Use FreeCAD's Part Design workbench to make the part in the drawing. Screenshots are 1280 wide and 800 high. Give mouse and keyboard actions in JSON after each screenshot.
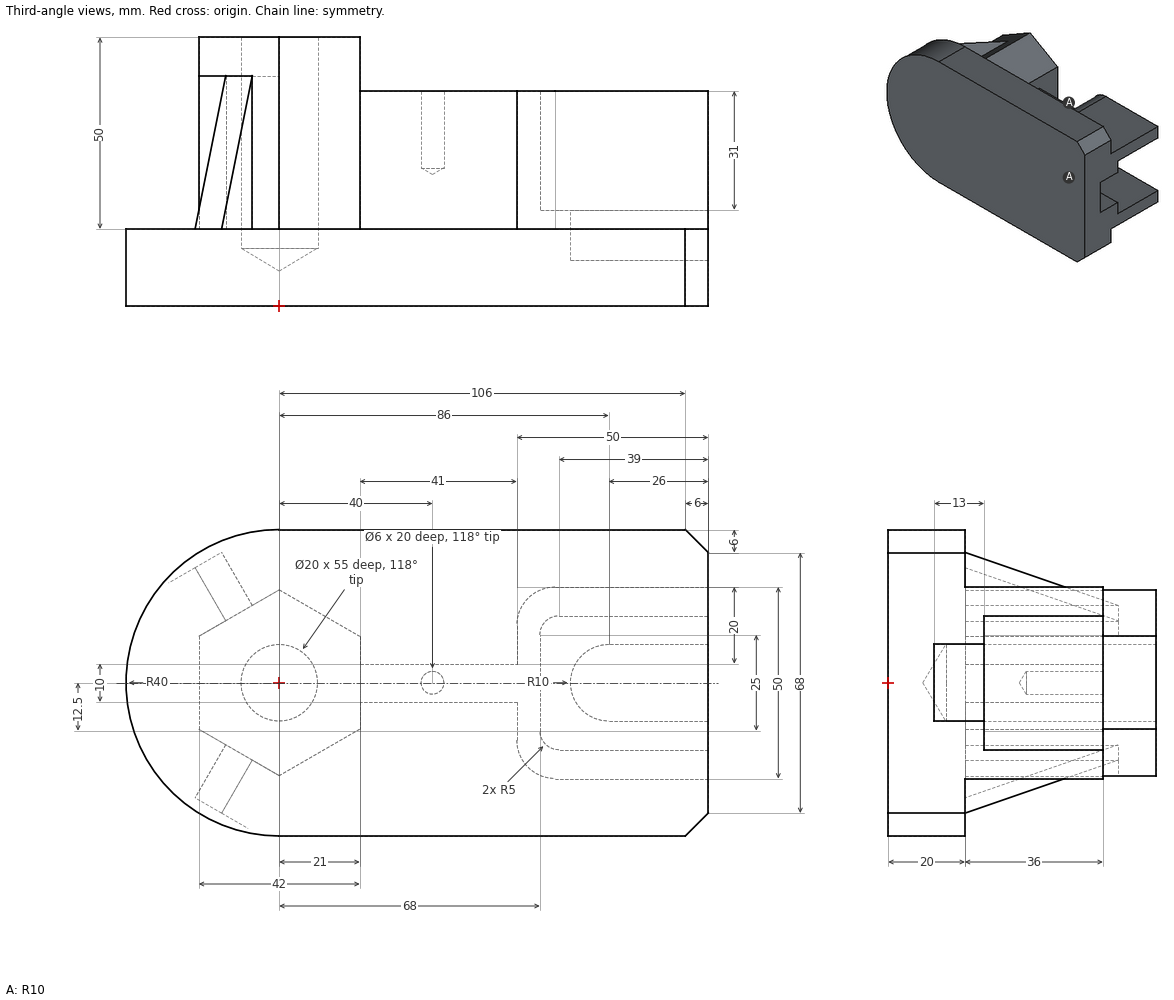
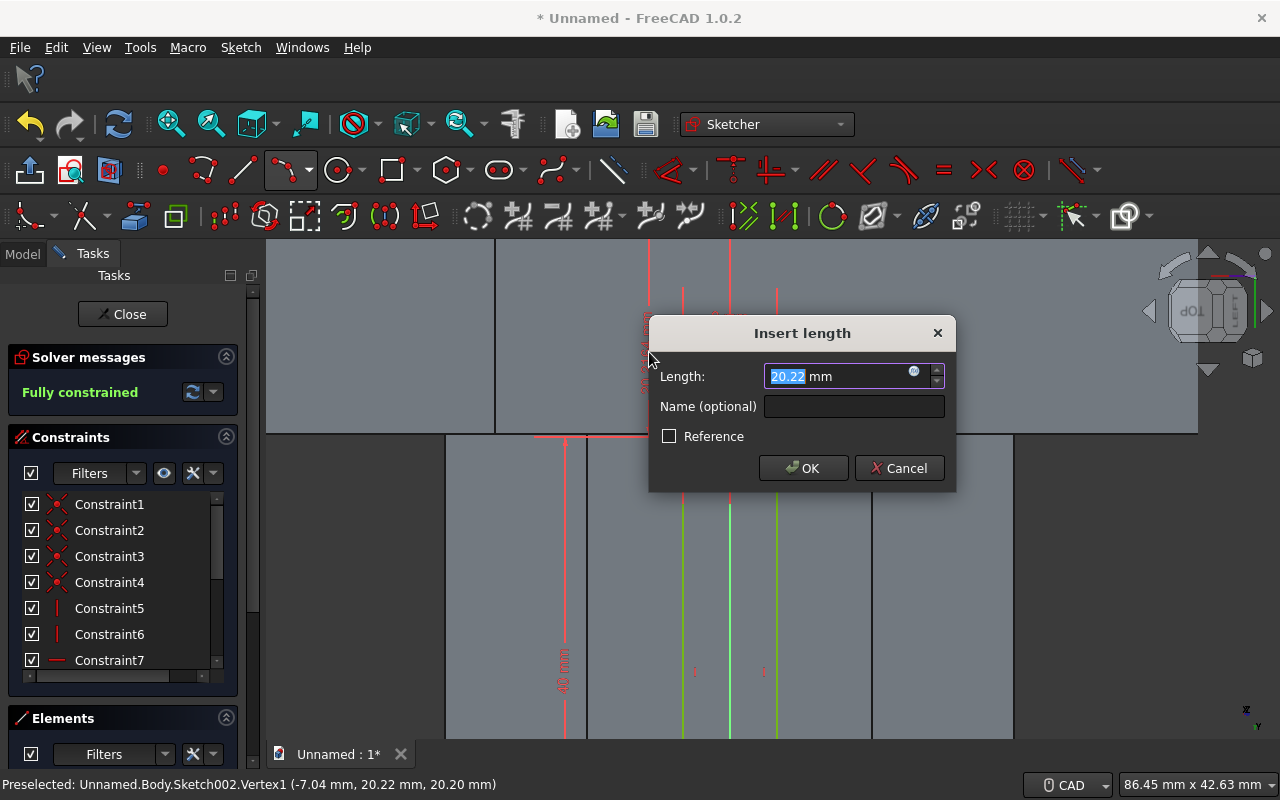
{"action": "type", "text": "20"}
{"action": "key", "text": "Return"}
{"action": "key", "text": "Escape"}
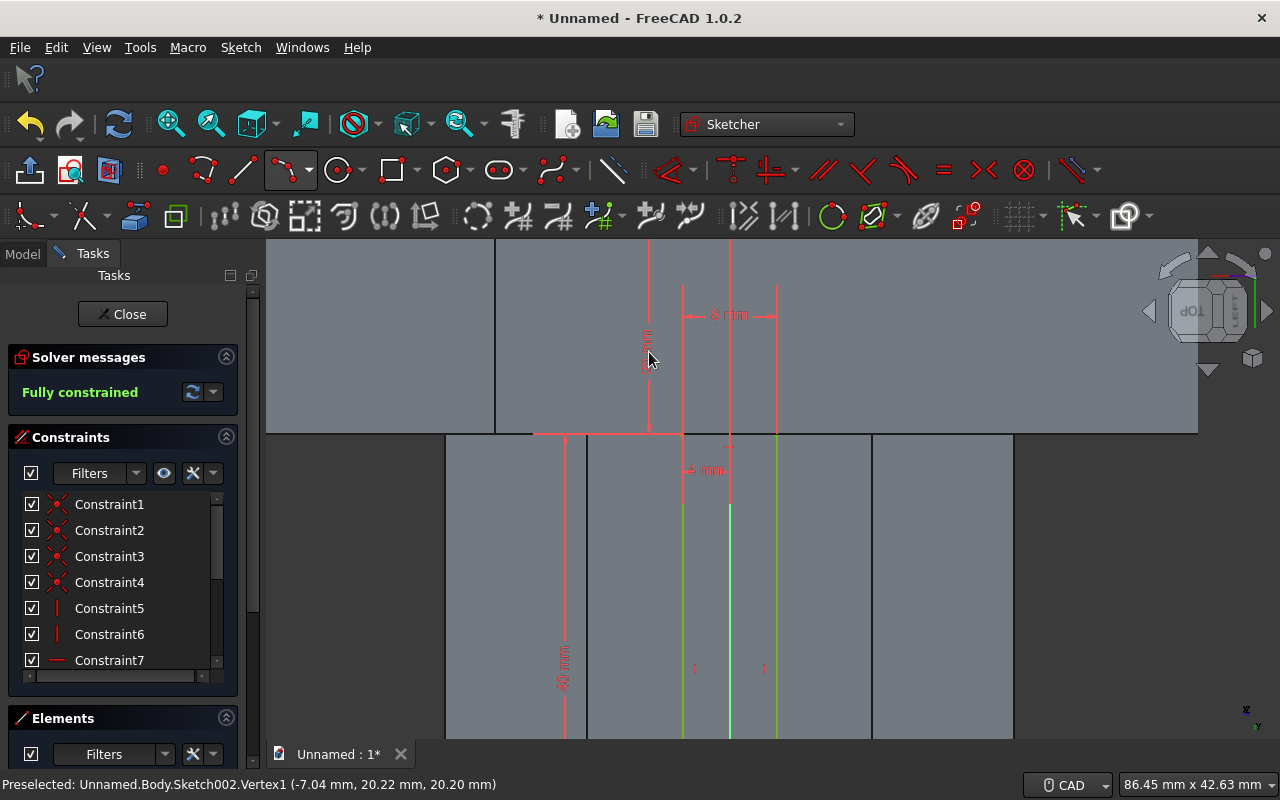
{"action": "left_click", "coordinate": [123, 314]}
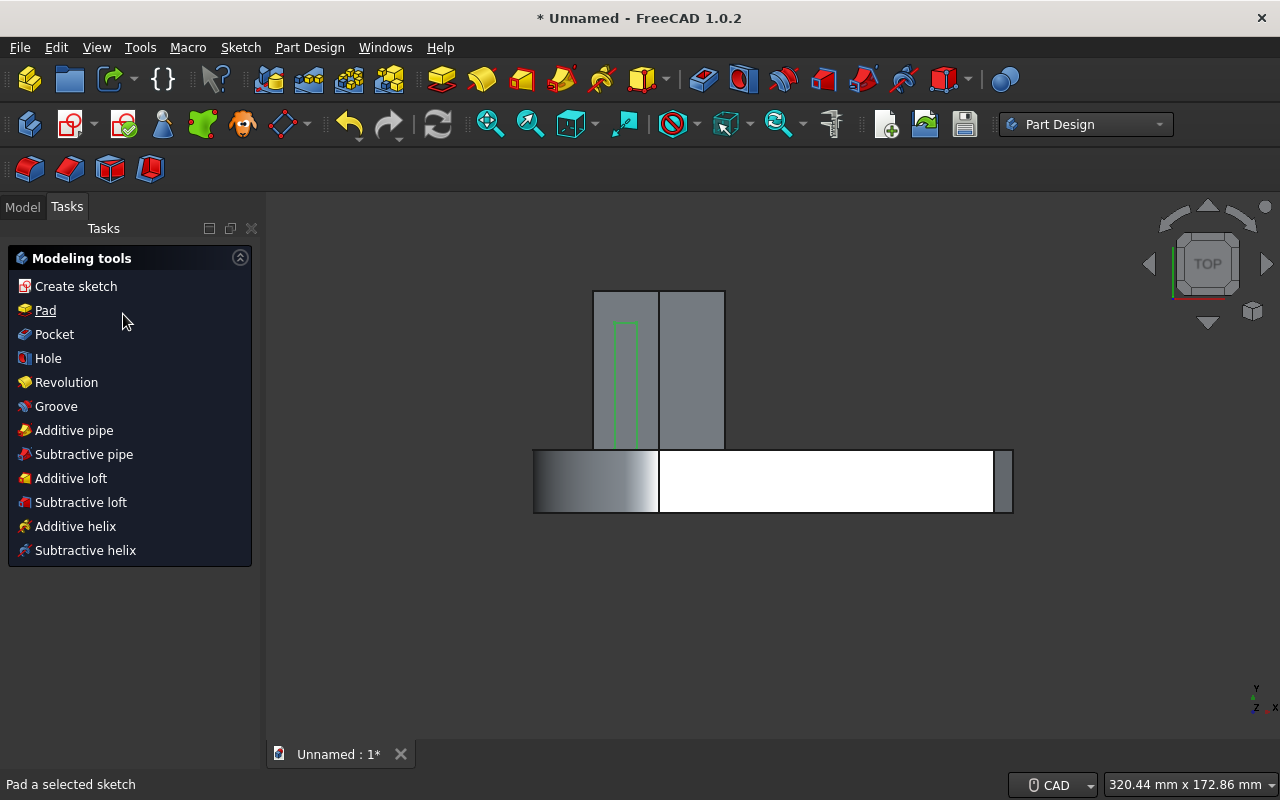
{"action": "left_click", "coordinate": [442, 80]}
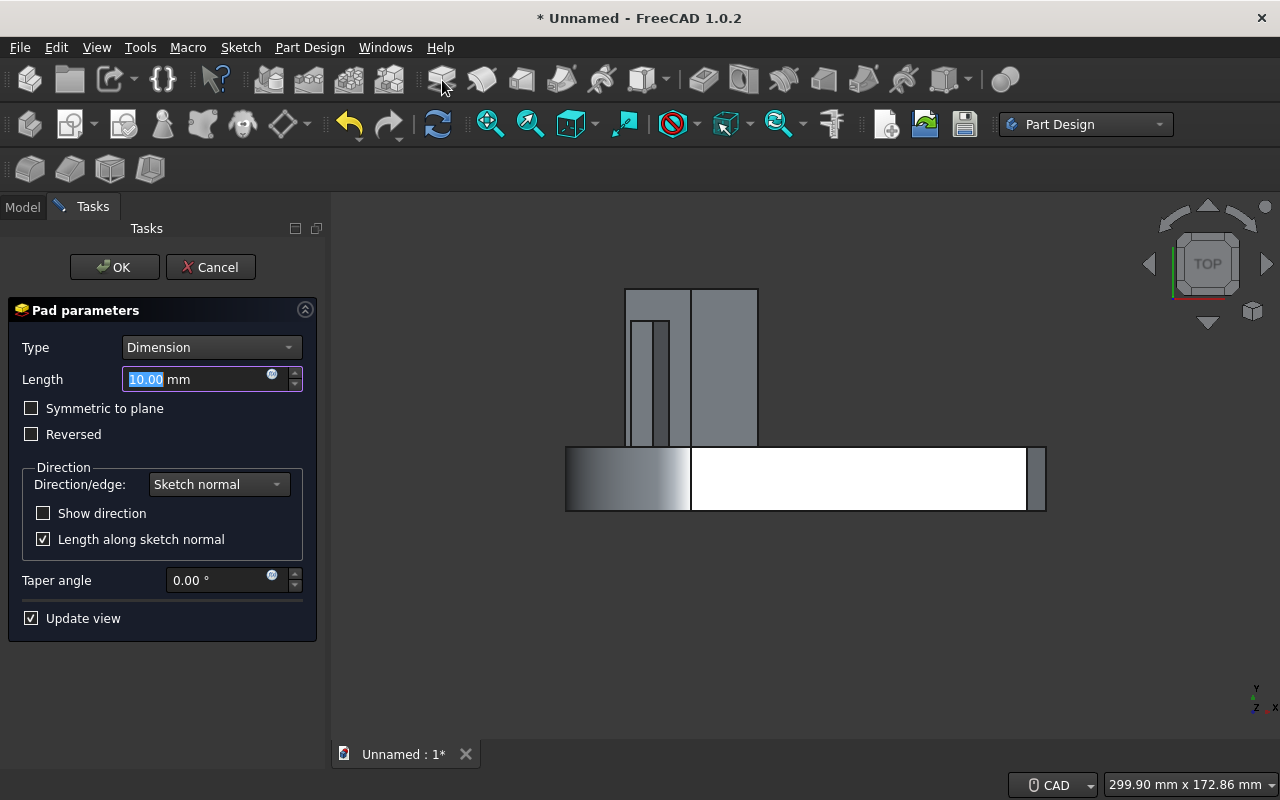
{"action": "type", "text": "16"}
{"action": "key", "text": "Tab"}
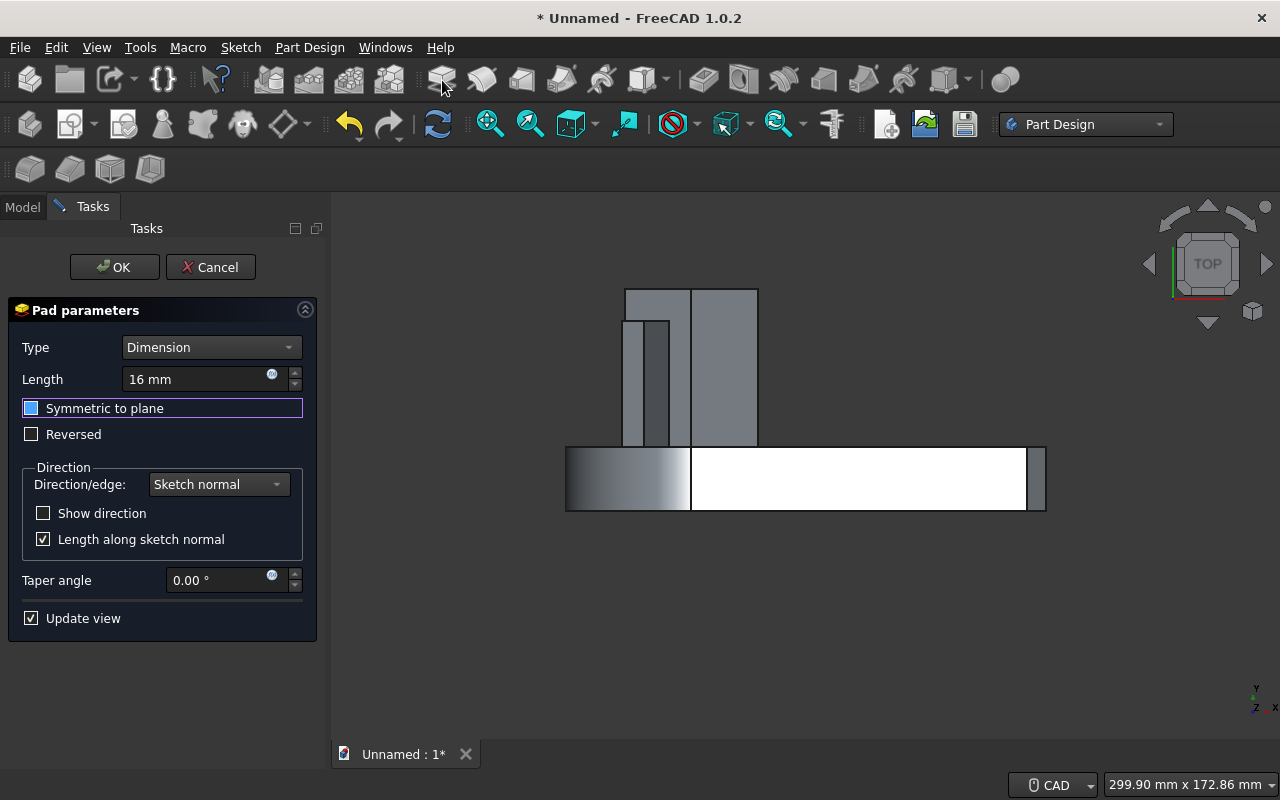
{"action": "left_click", "coordinate": [115, 267]}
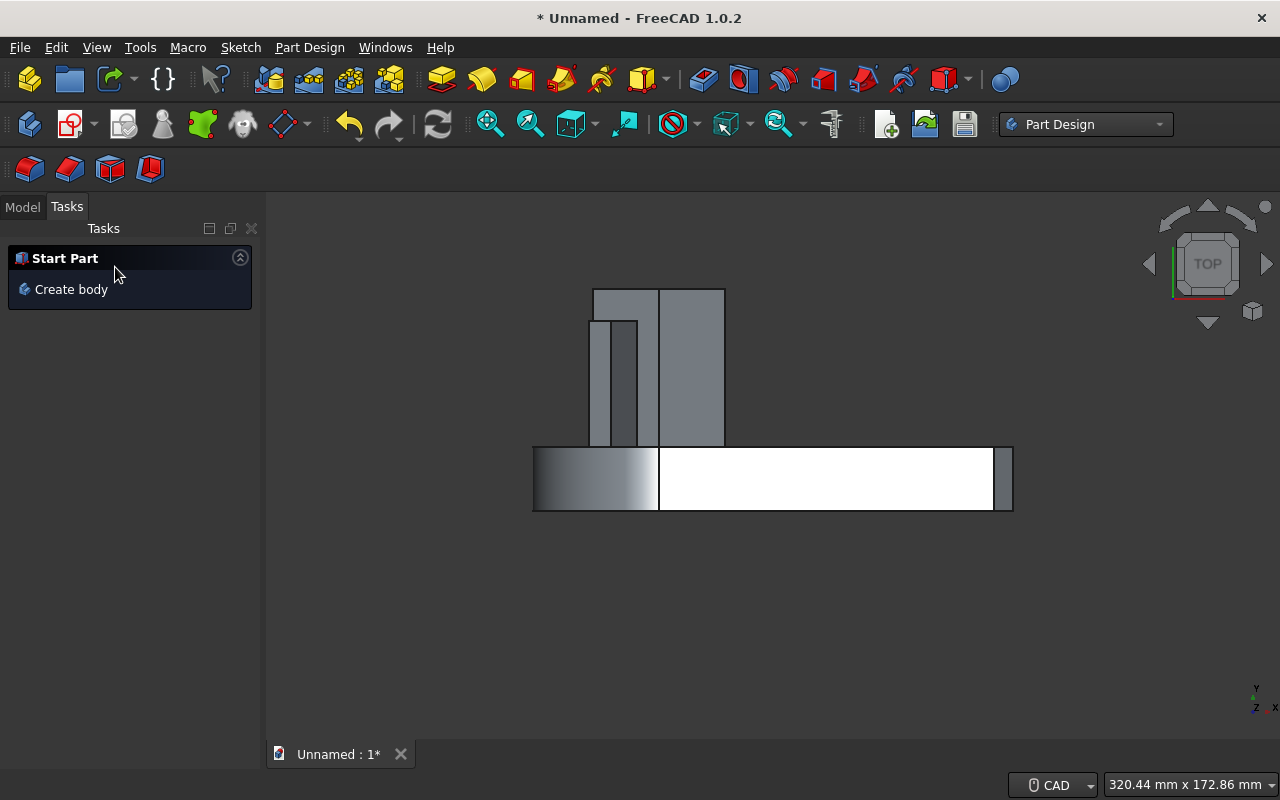
{"action": "left_click", "coordinate": [624, 365]}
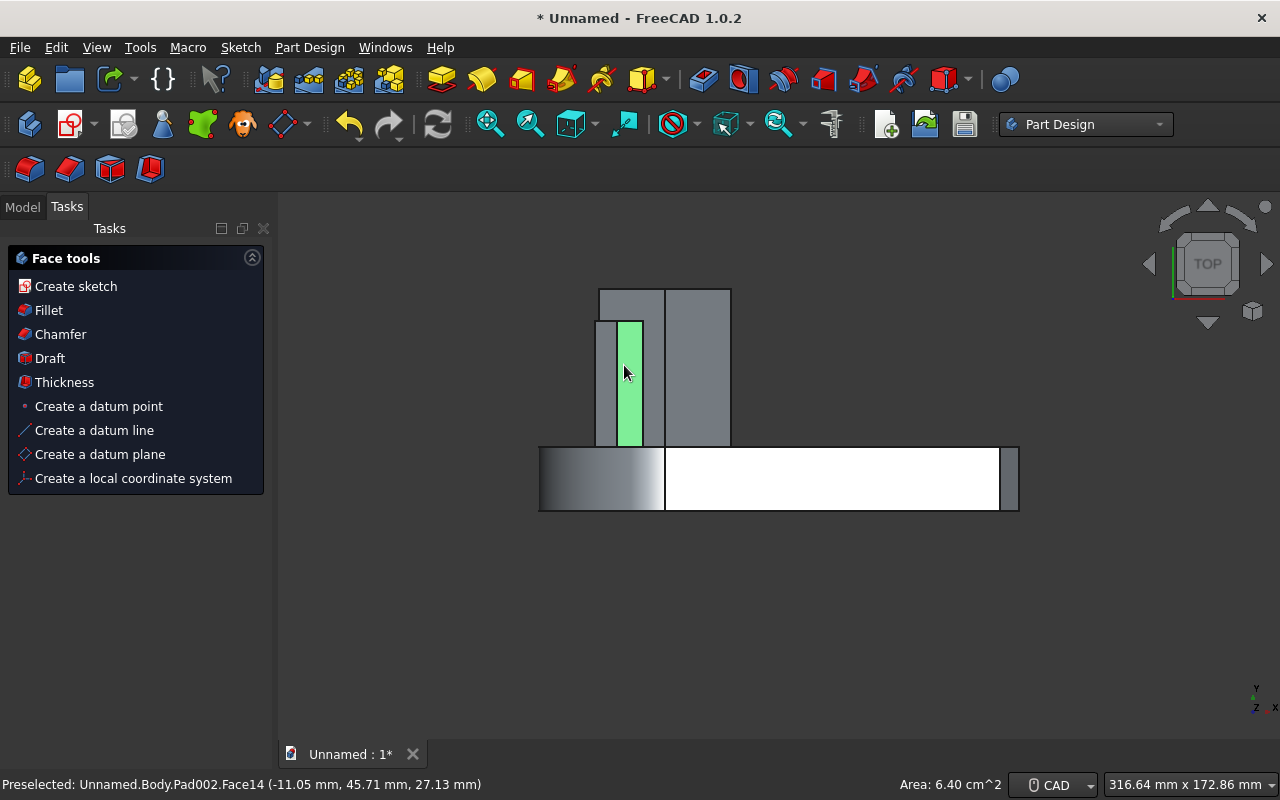
{"action": "left_click", "coordinate": [70, 124]}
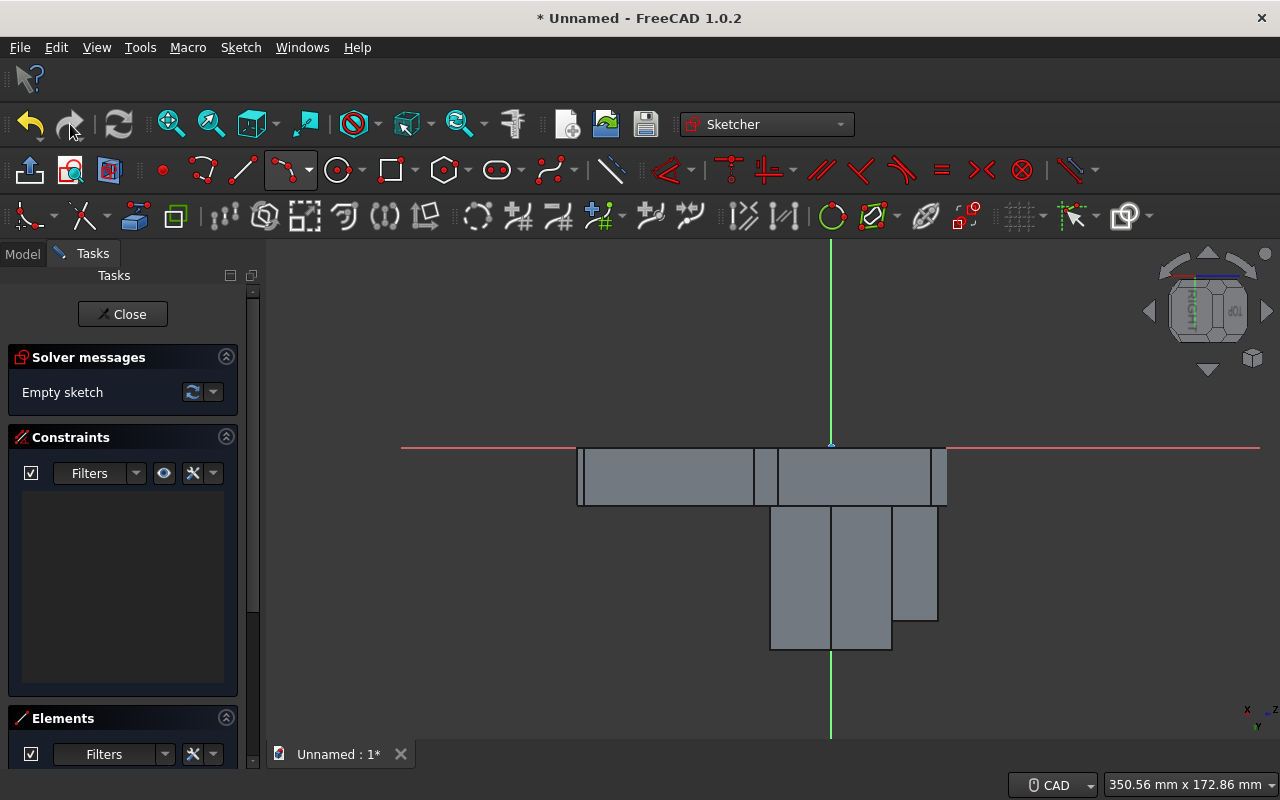
{"action": "scroll", "coordinate": [1103, 590], "scroll_direction": "up", "scroll_amount": 3}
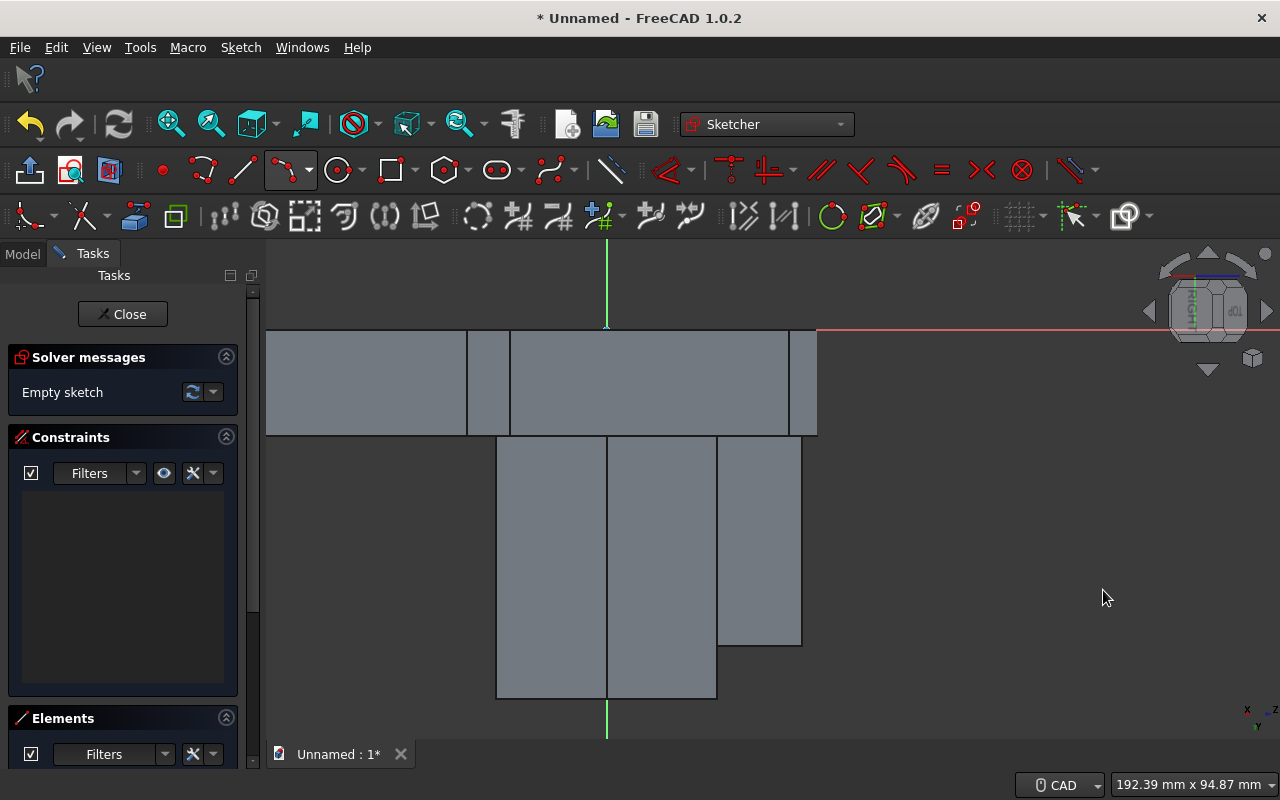
{"action": "left_click", "coordinate": [204, 170]}